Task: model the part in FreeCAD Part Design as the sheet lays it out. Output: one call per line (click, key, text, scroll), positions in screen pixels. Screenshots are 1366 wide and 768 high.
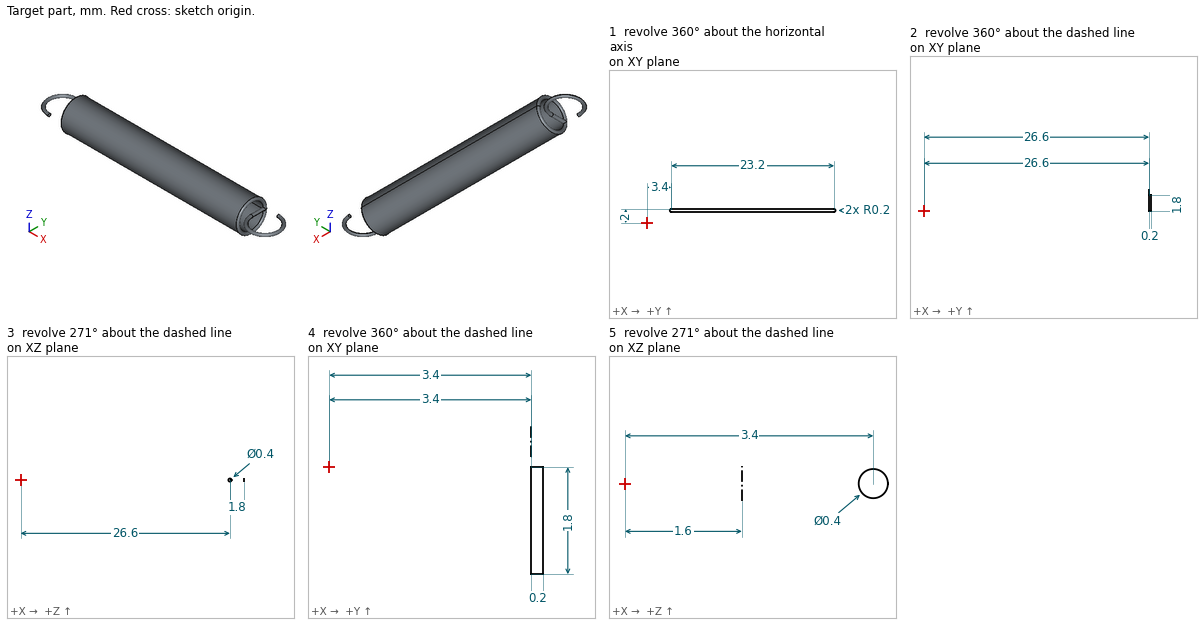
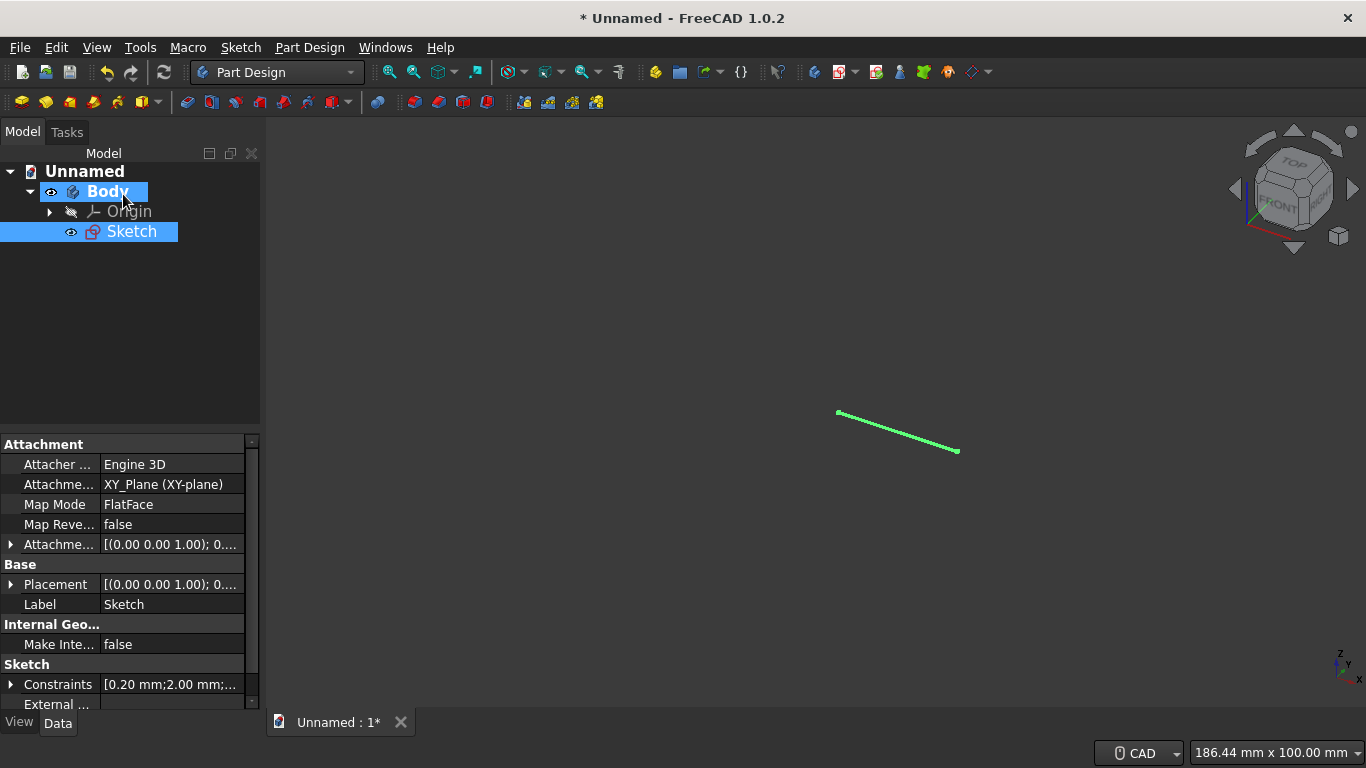
click(46, 102)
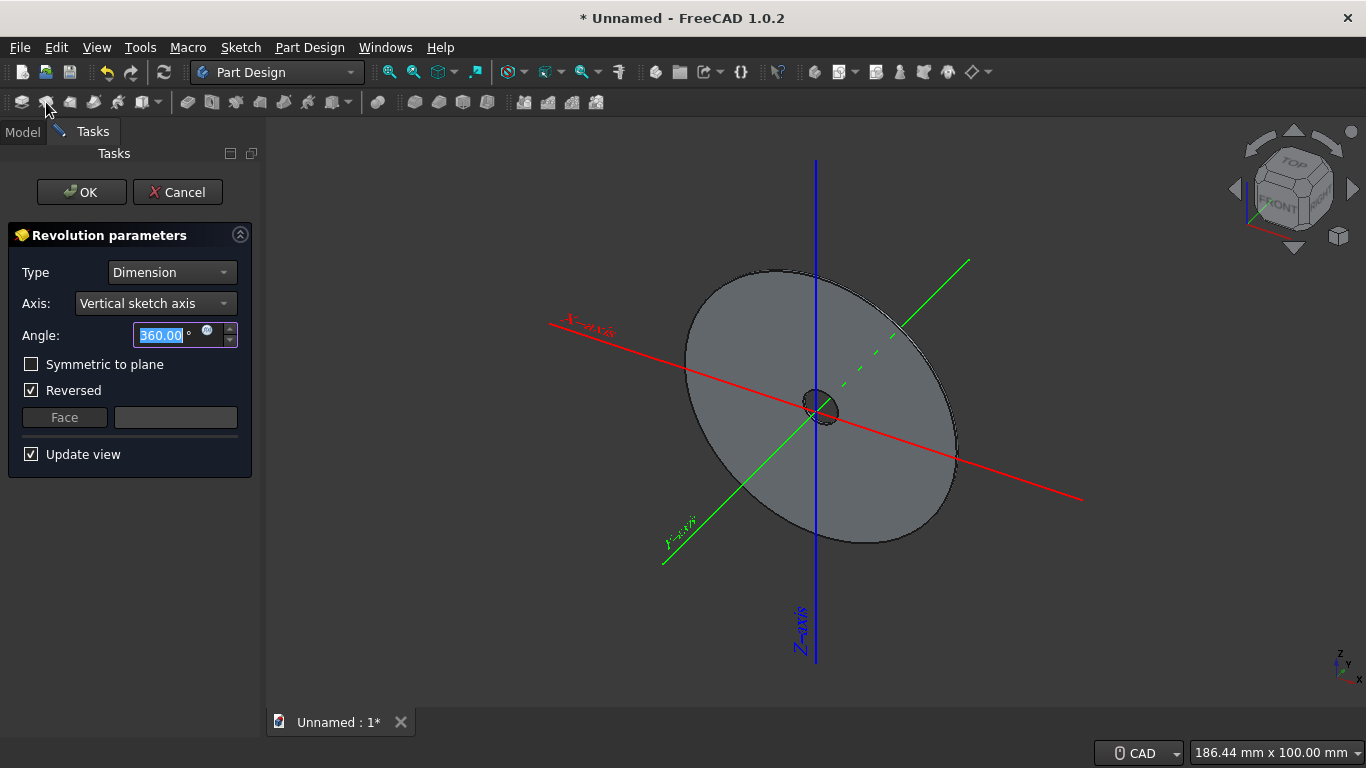
click(156, 304)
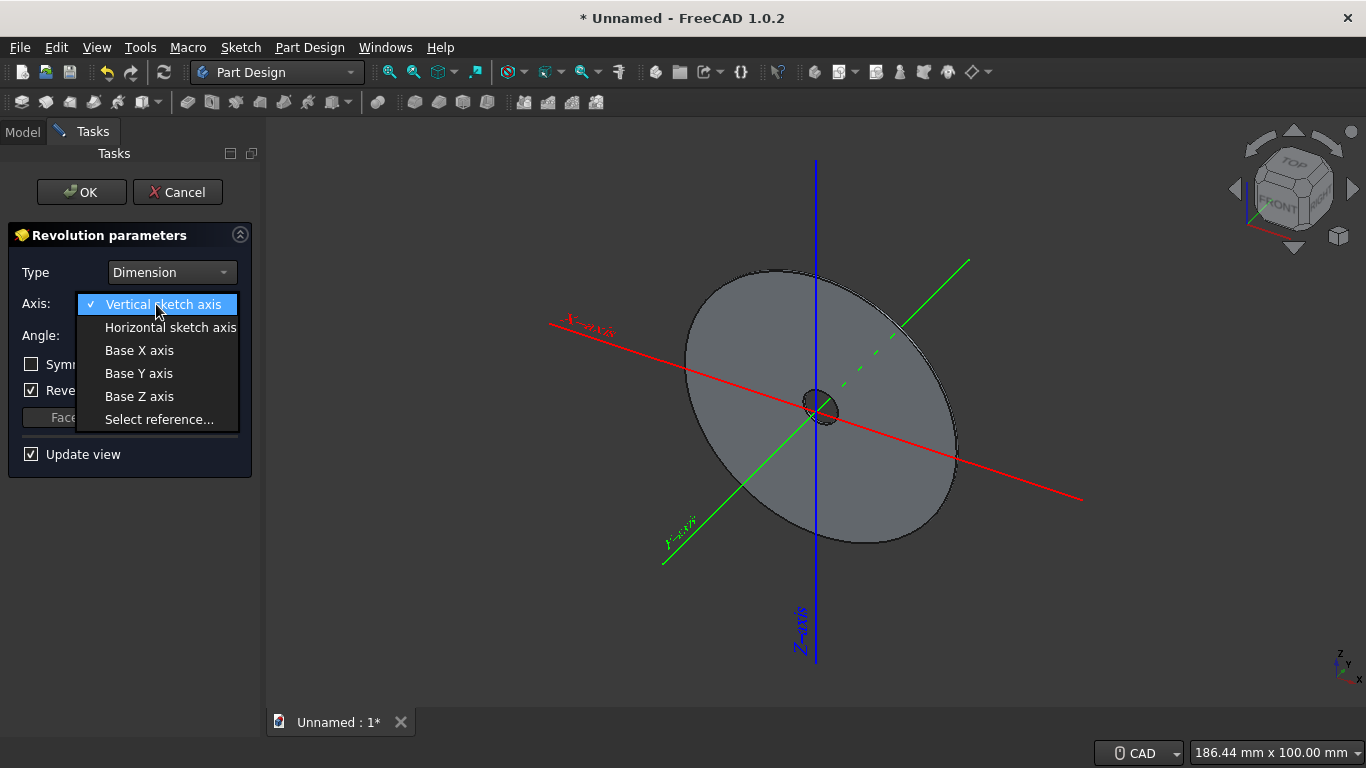
click(156, 328)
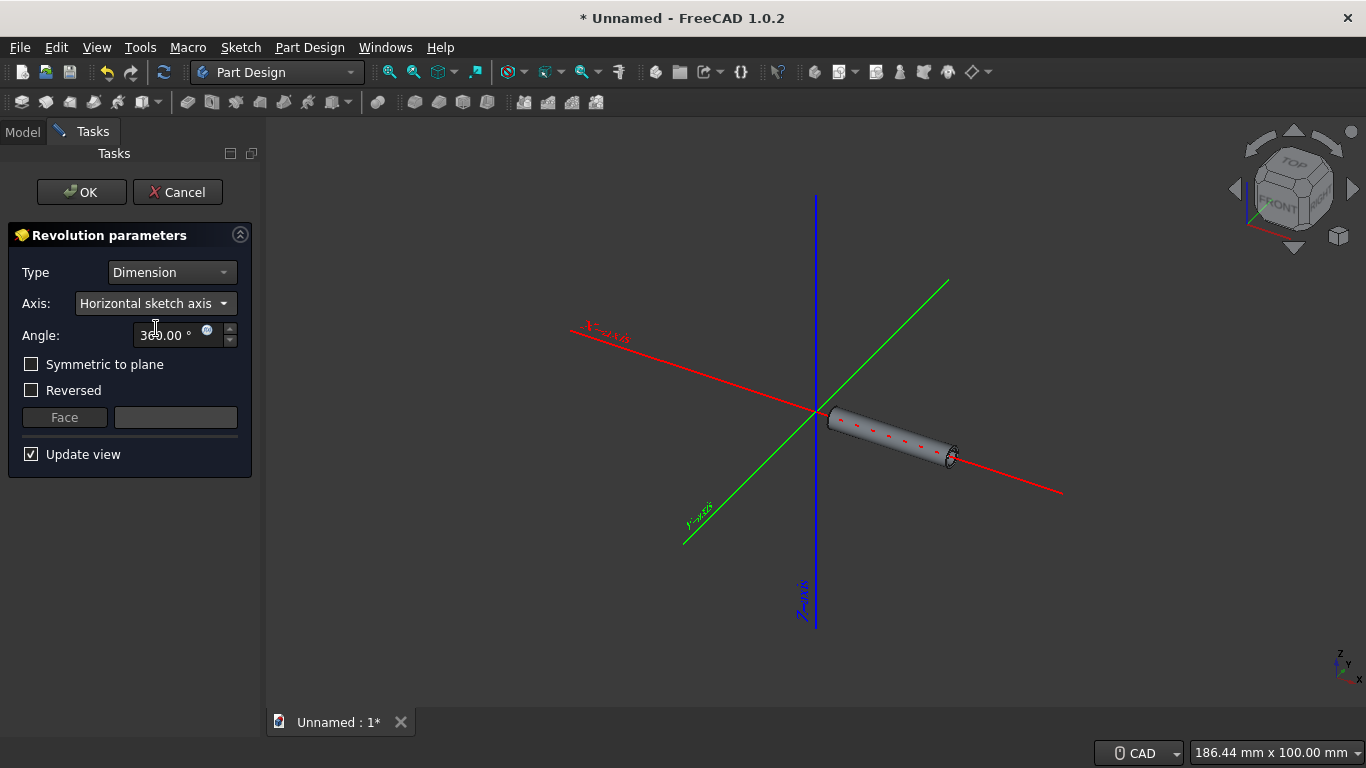
click(82, 192)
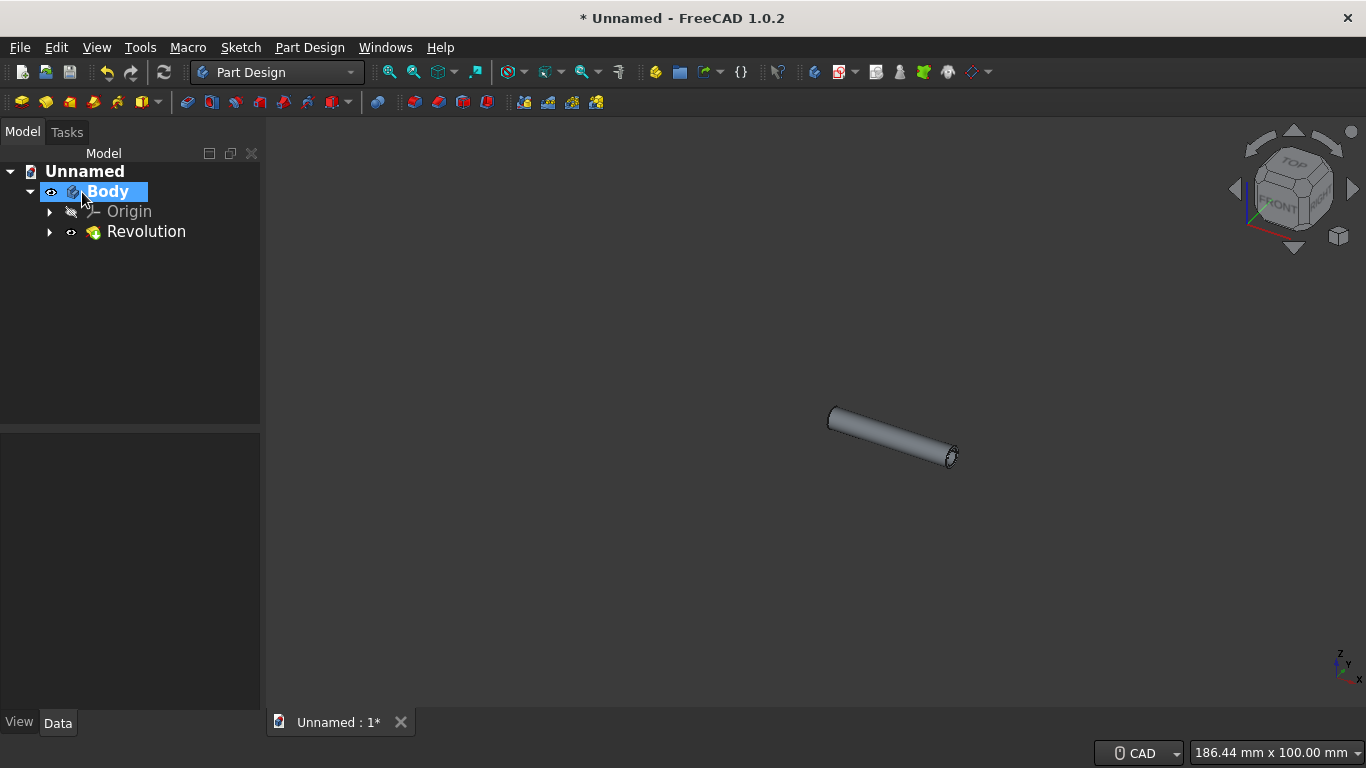
click(390, 72)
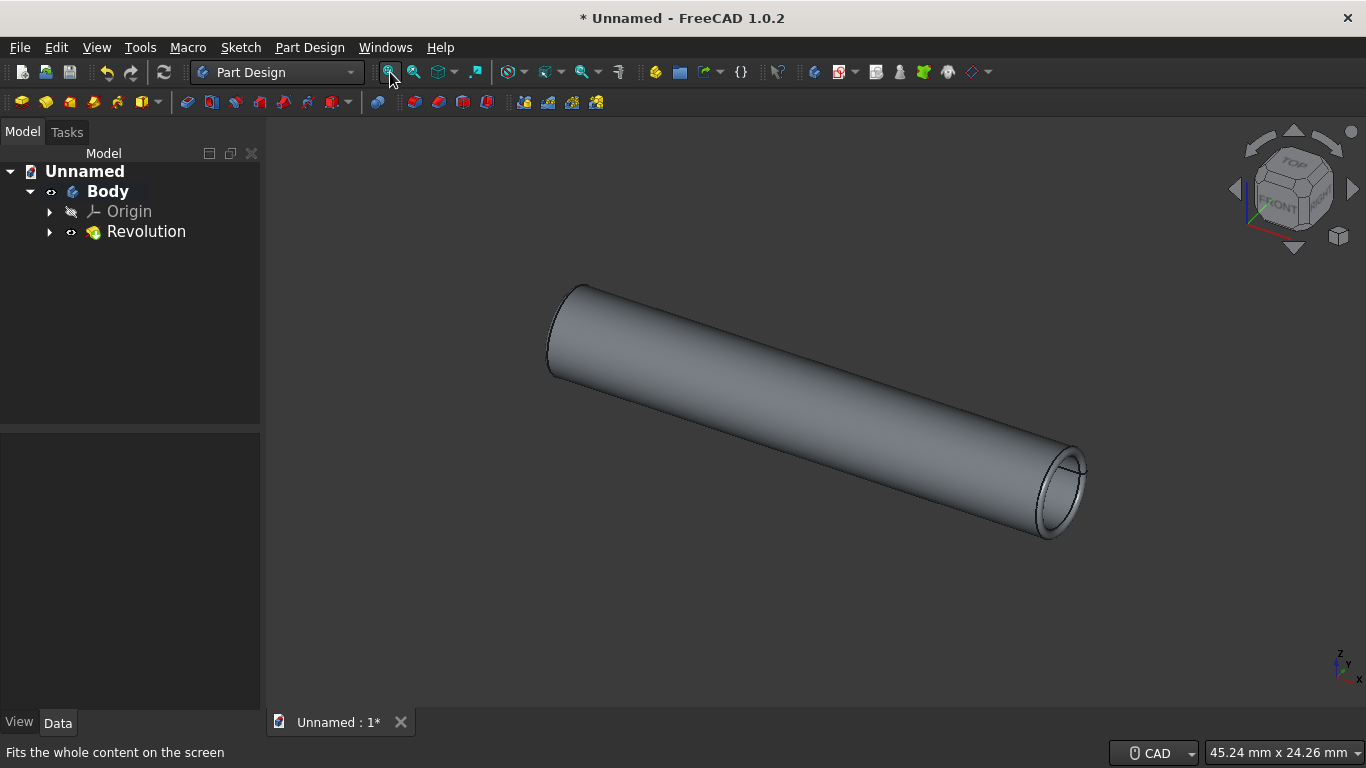
click(840, 72)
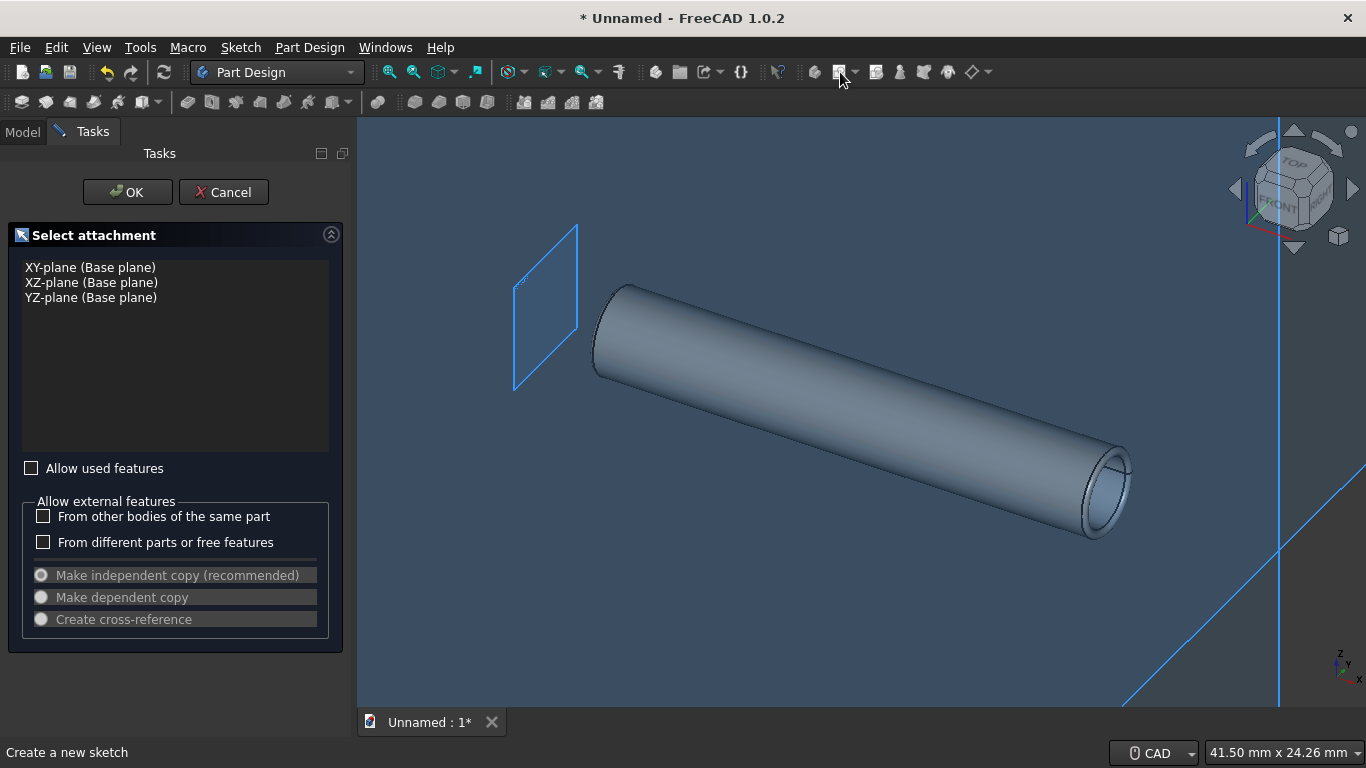
click(82, 268)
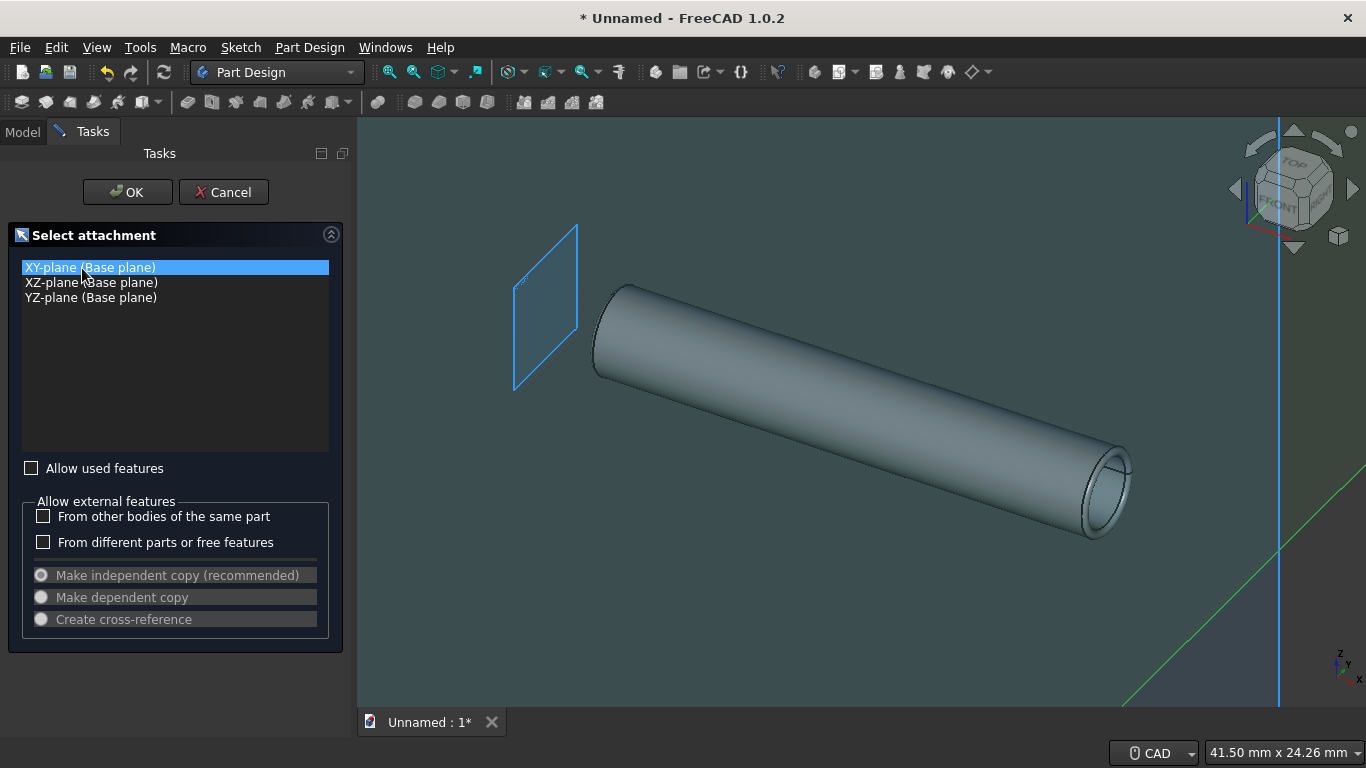
click(128, 192)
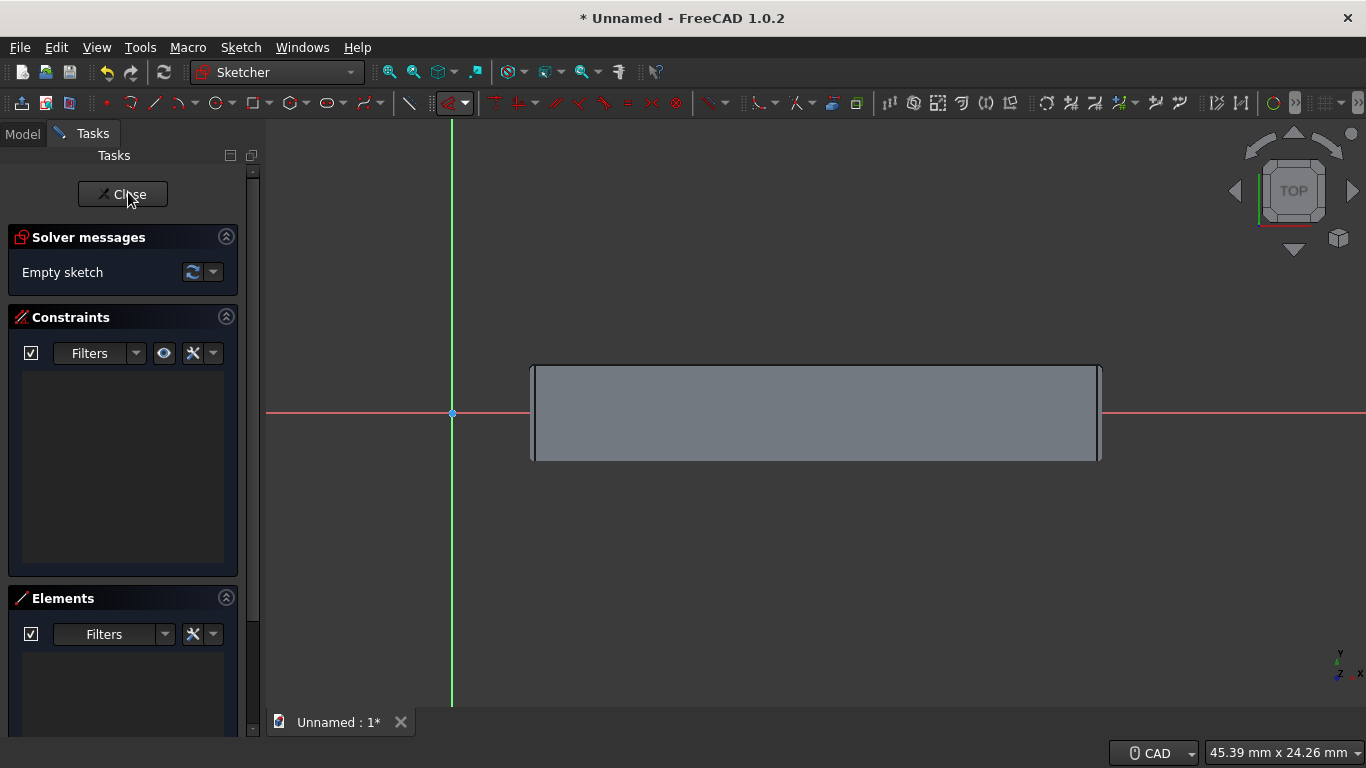
click(70, 104)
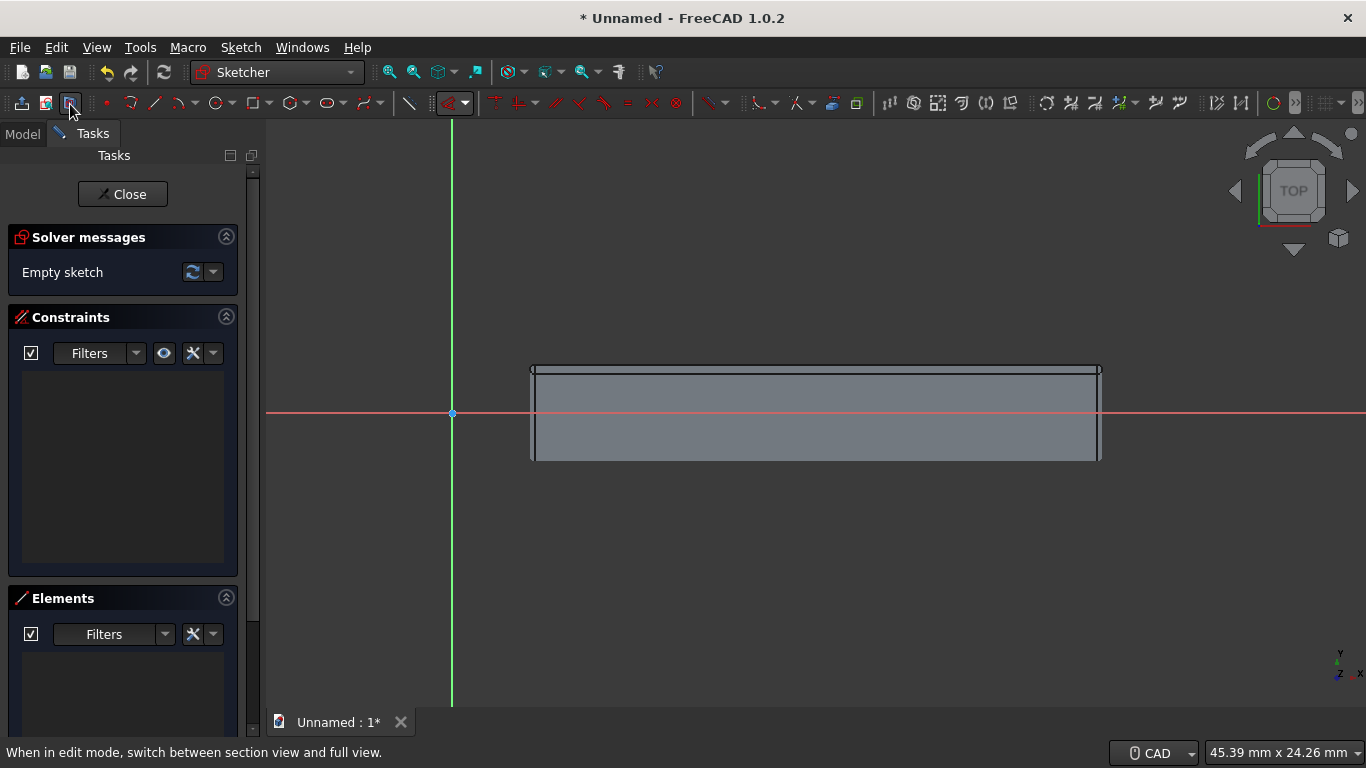
scroll(1169, 377, up, 9)